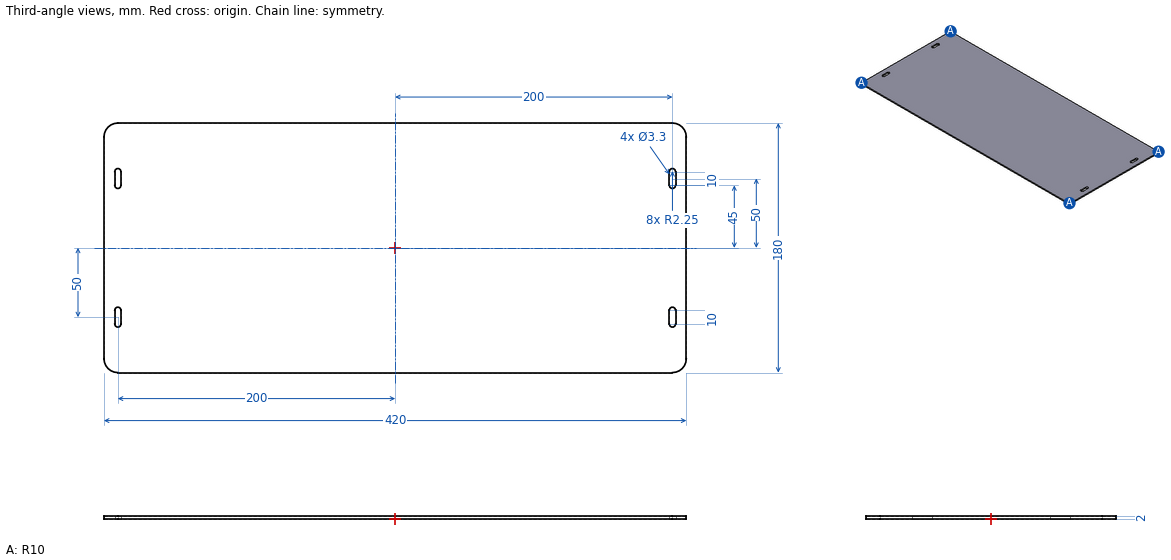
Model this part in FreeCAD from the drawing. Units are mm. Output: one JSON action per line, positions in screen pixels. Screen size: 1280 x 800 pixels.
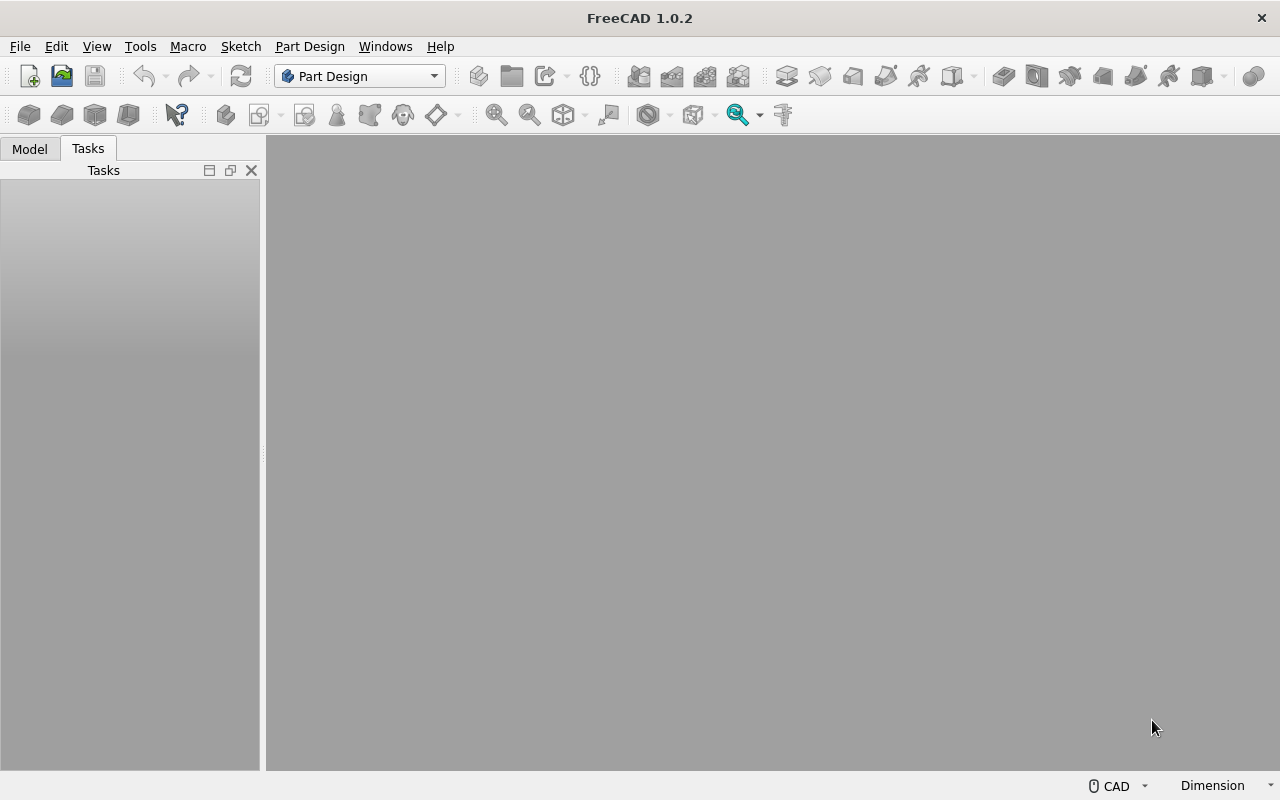
{"action": "left_click", "coordinate": [29, 76]}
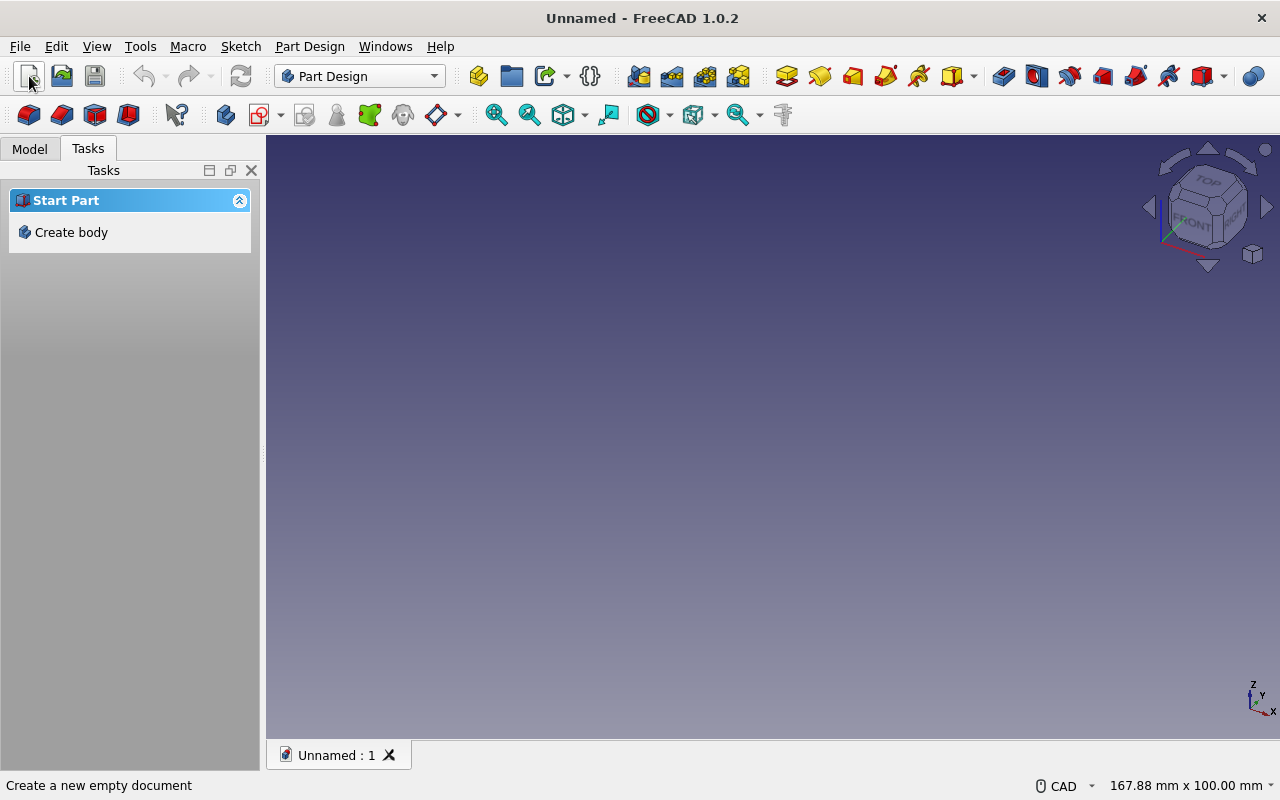
{"action": "left_click", "coordinate": [258, 116]}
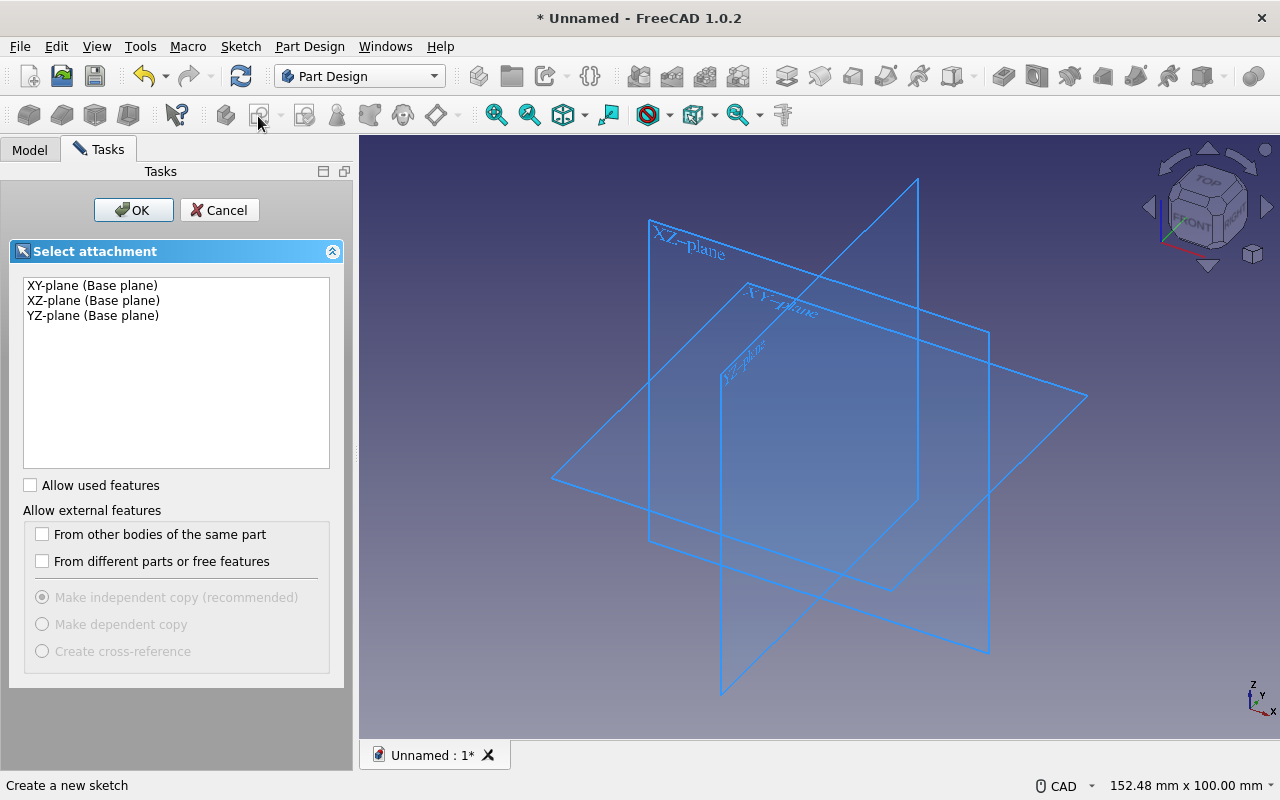
{"action": "left_click", "coordinate": [84, 286]}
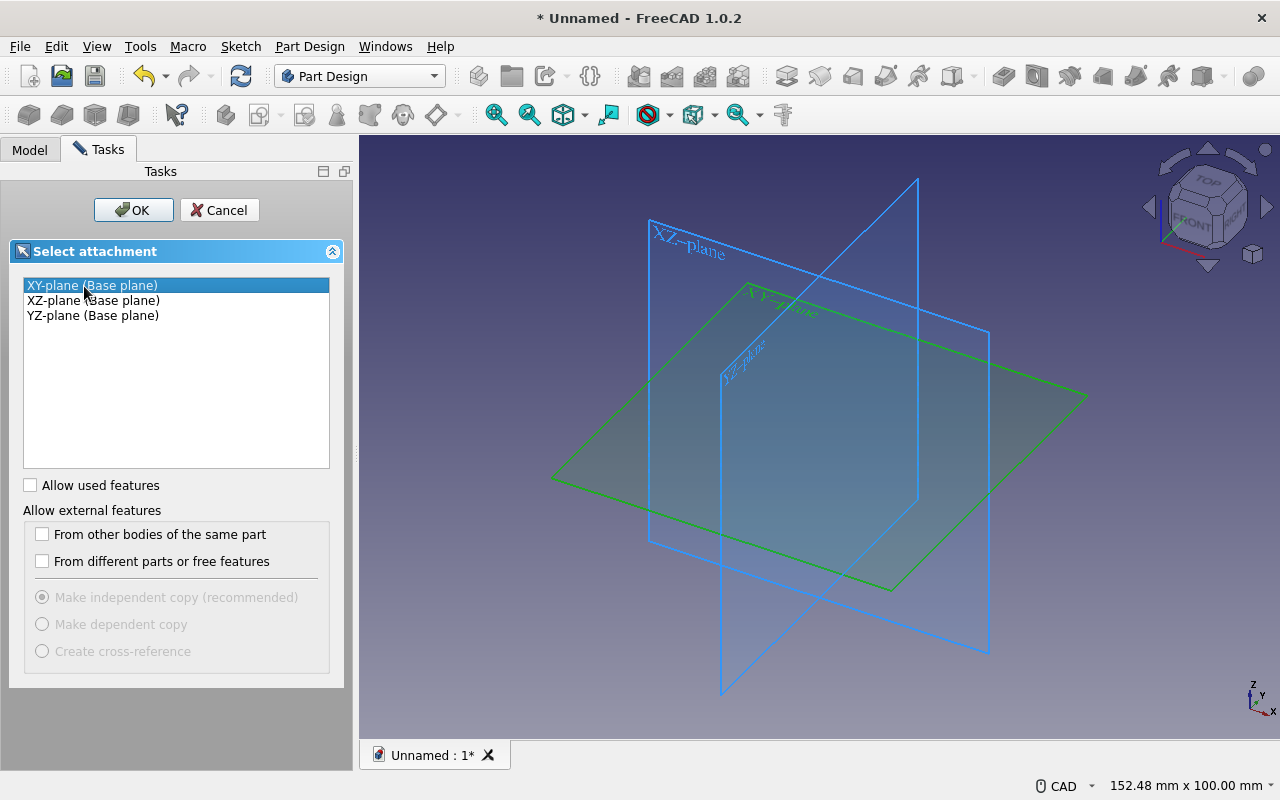
{"action": "left_click", "coordinate": [134, 210]}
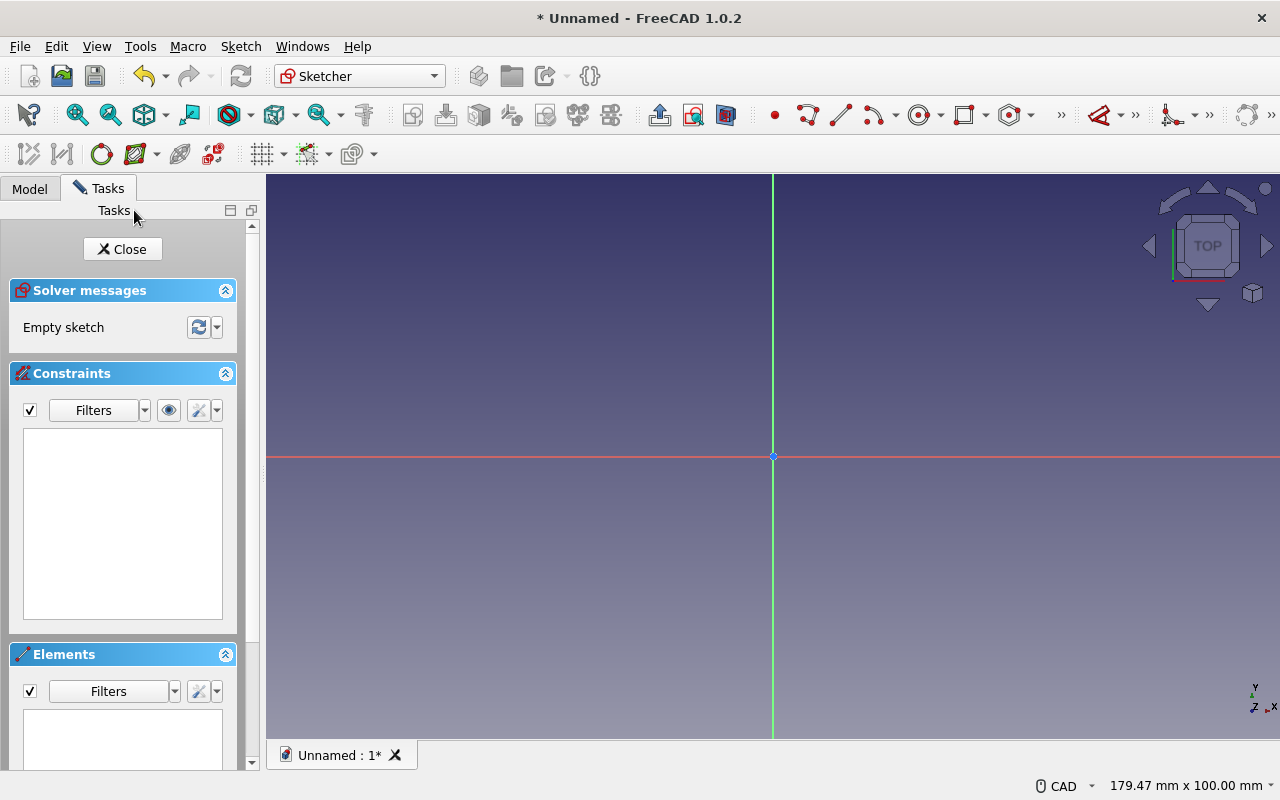
{"action": "scroll", "coordinate": [682, 456], "scroll_direction": "down", "scroll_amount": 7}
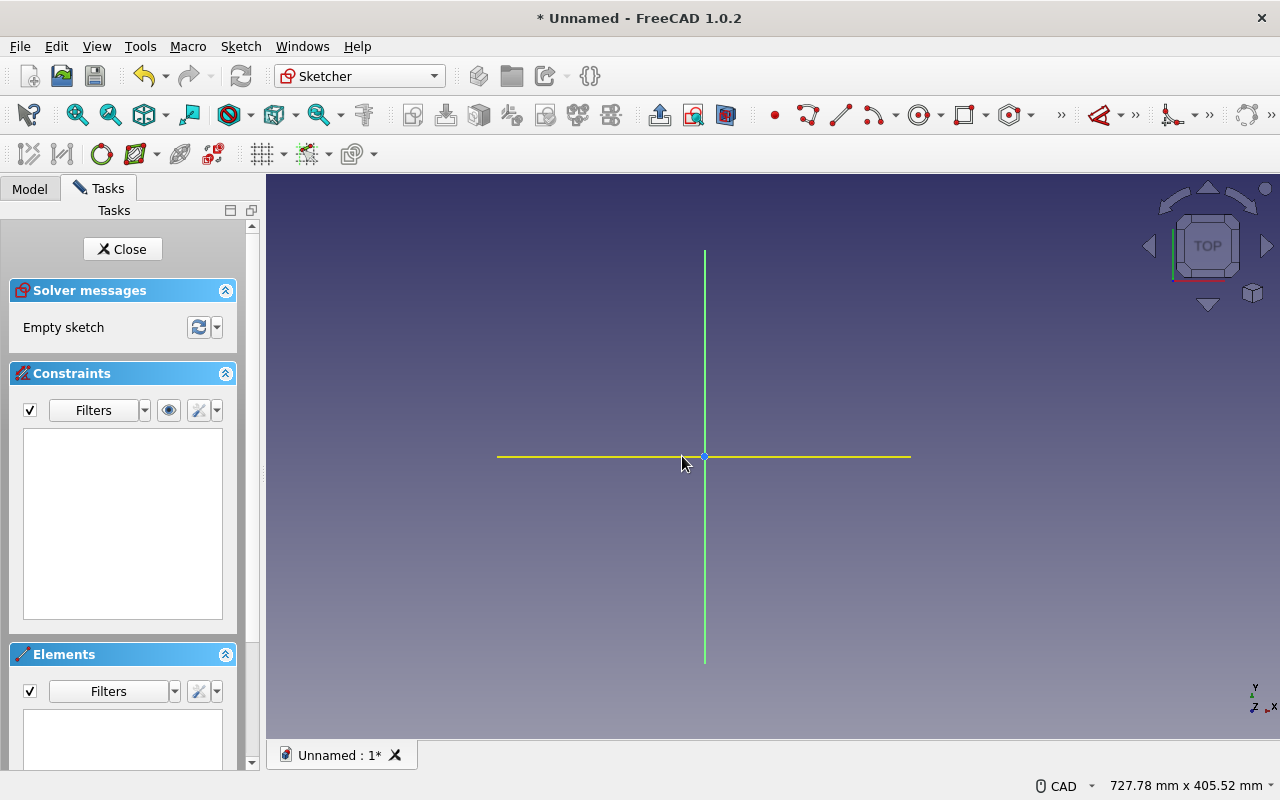
{"action": "key", "text": "g v"}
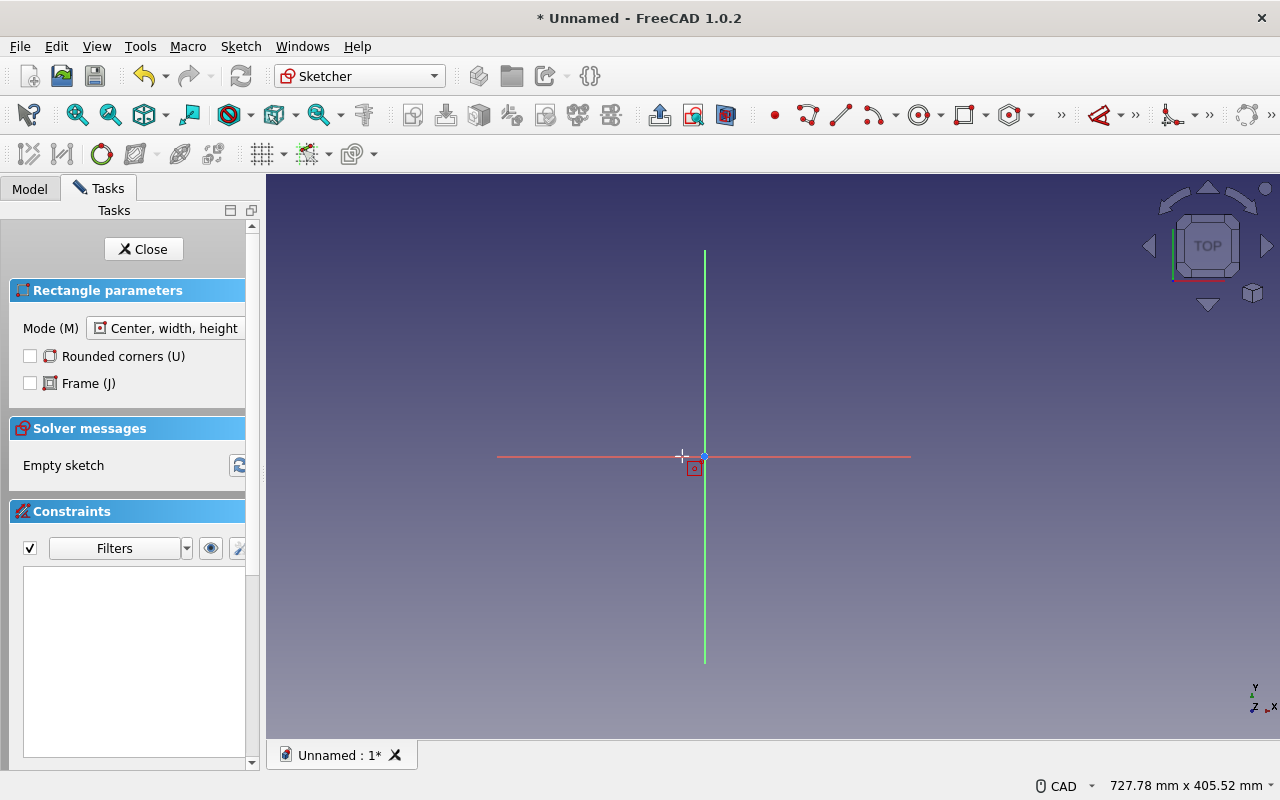
{"action": "left_click", "coordinate": [705, 456]}
{"action": "mouse_move", "coordinate": [997, 331]}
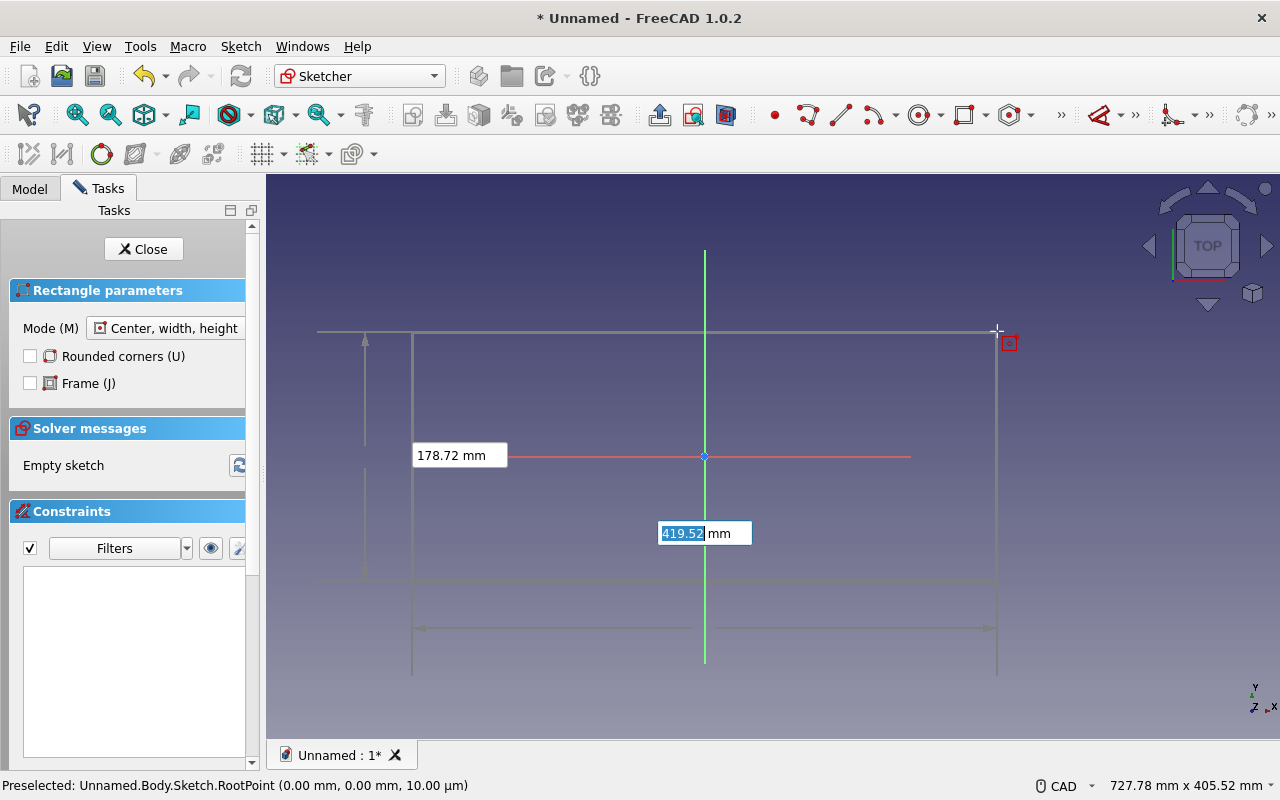
{"action": "type", "text": "420"}
{"action": "key", "text": "Tab"}
{"action": "type", "text": "180"}
{"action": "key", "text": "Return"}
{"action": "key", "text": "Escape"}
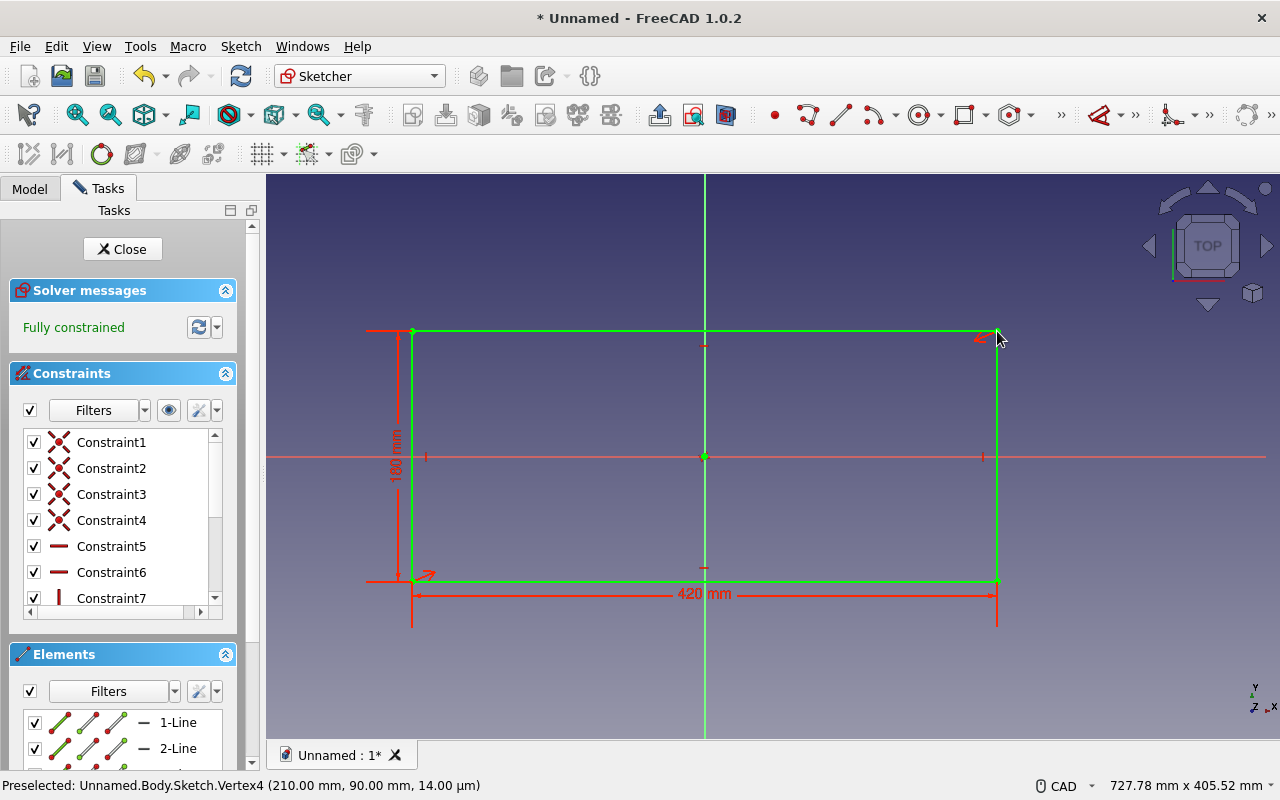
{"action": "left_click", "coordinate": [123, 249]}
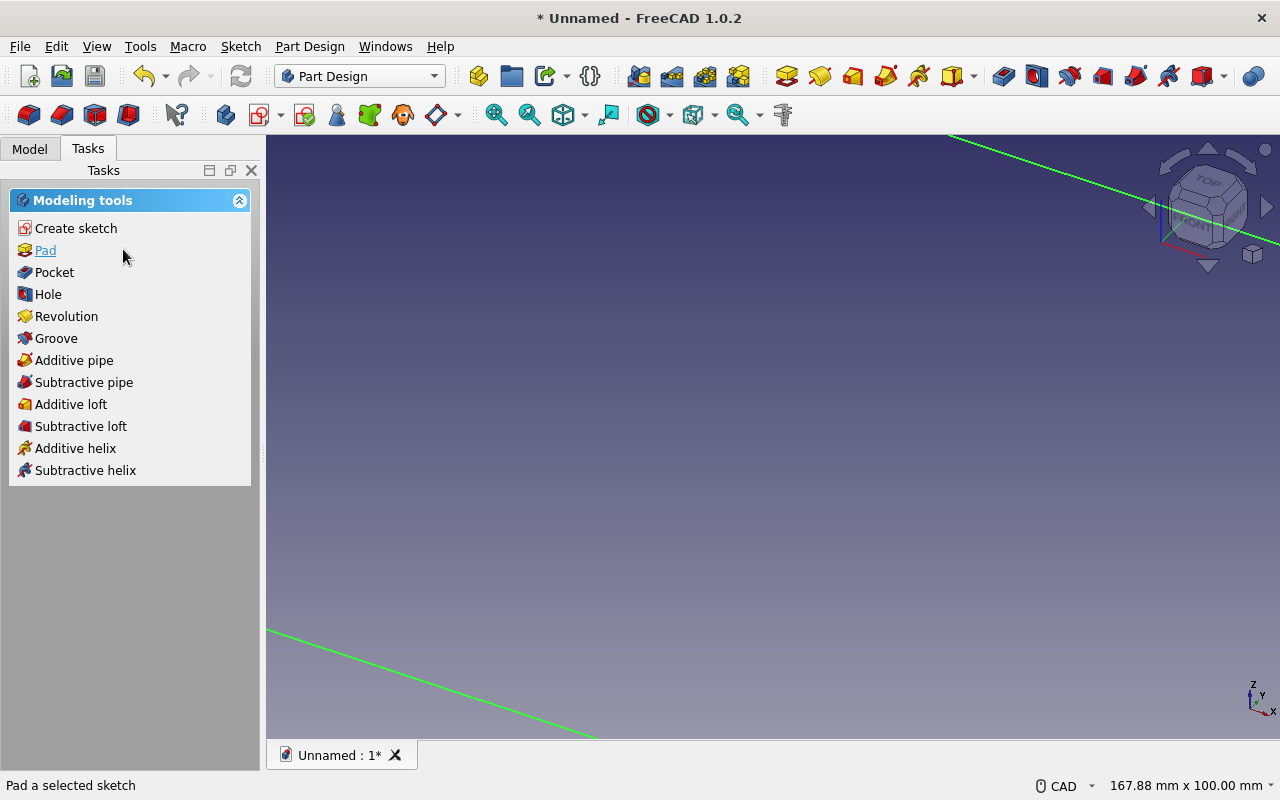
{"action": "left_click", "coordinate": [787, 76]}